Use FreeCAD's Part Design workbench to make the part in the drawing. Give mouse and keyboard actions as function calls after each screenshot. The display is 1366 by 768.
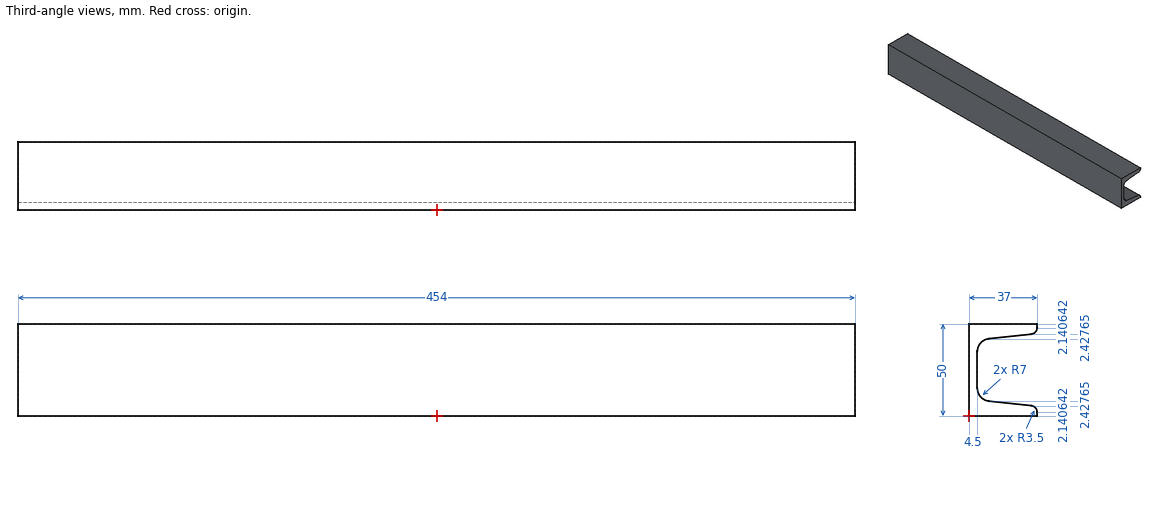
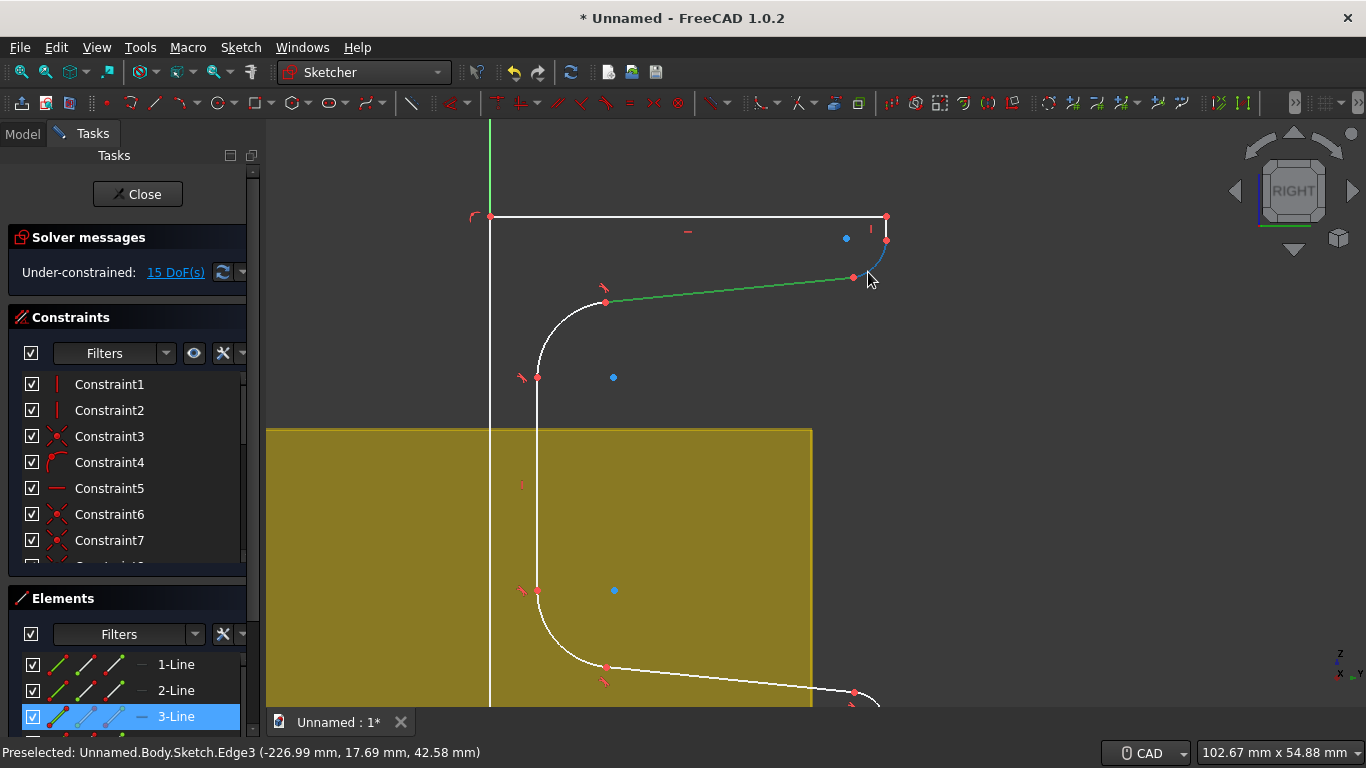
click(868, 272)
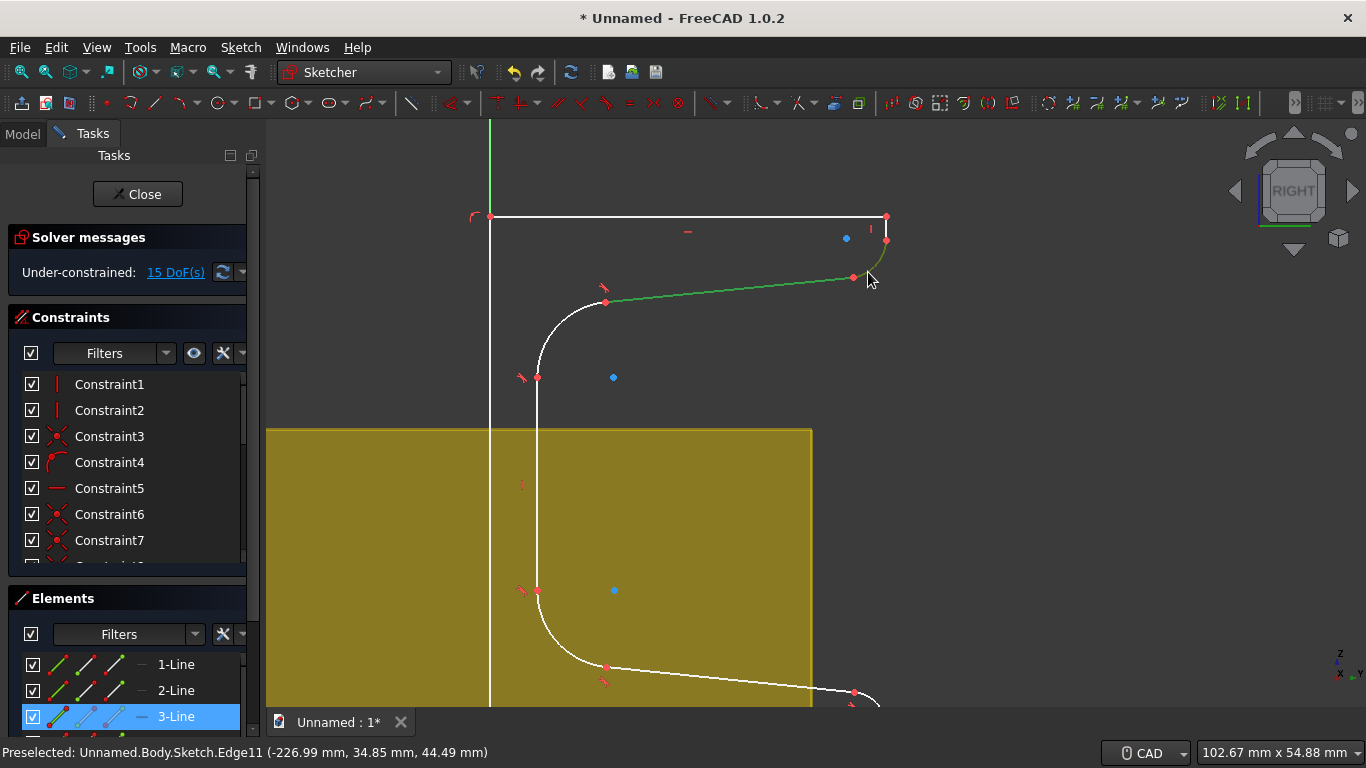
click(606, 104)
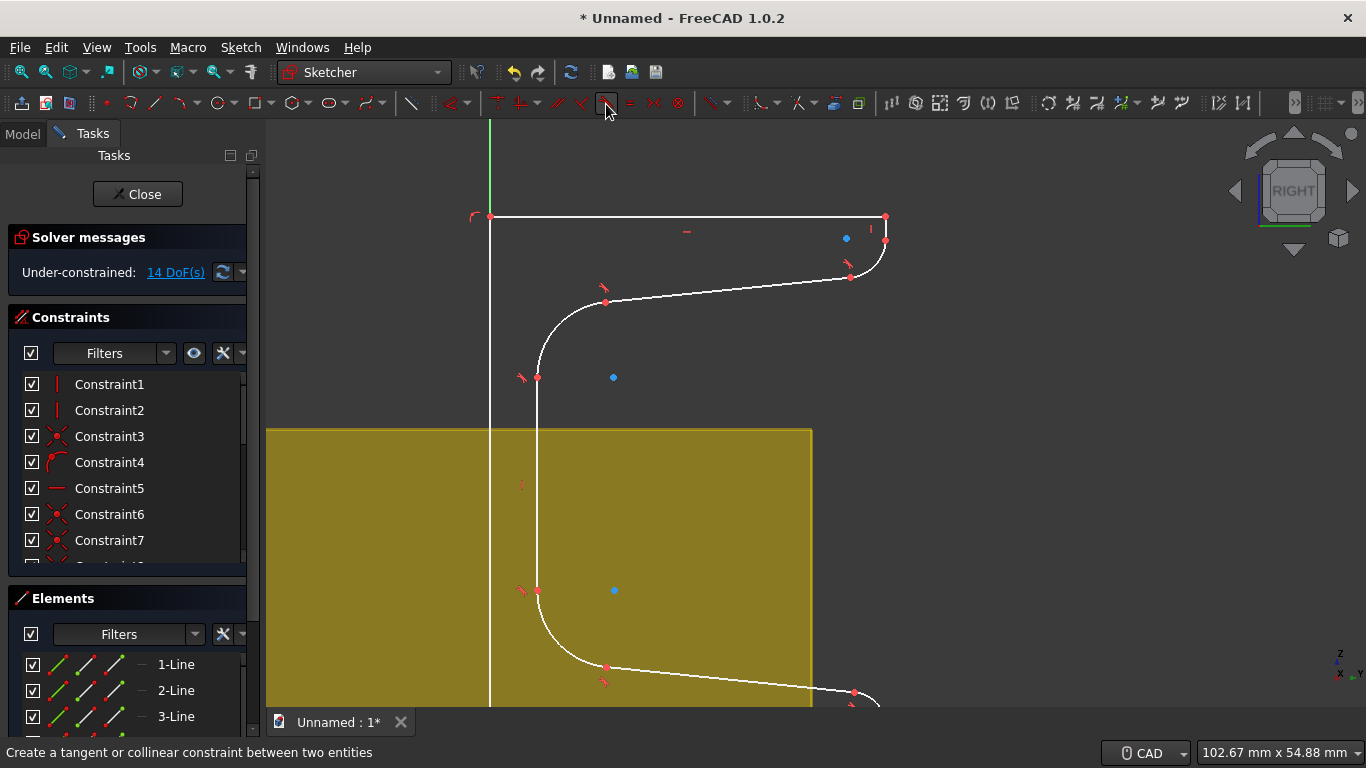
scroll(886, 231, up, 2)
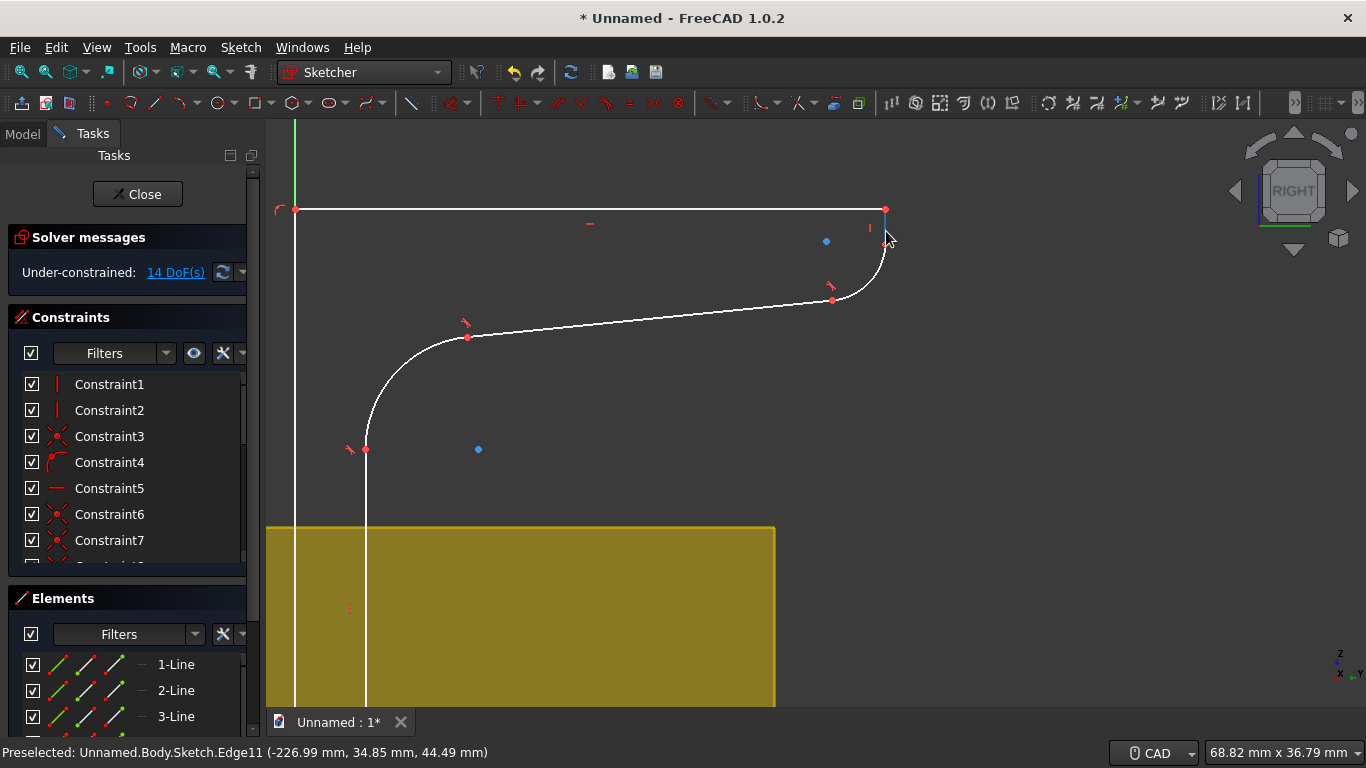
click(885, 231)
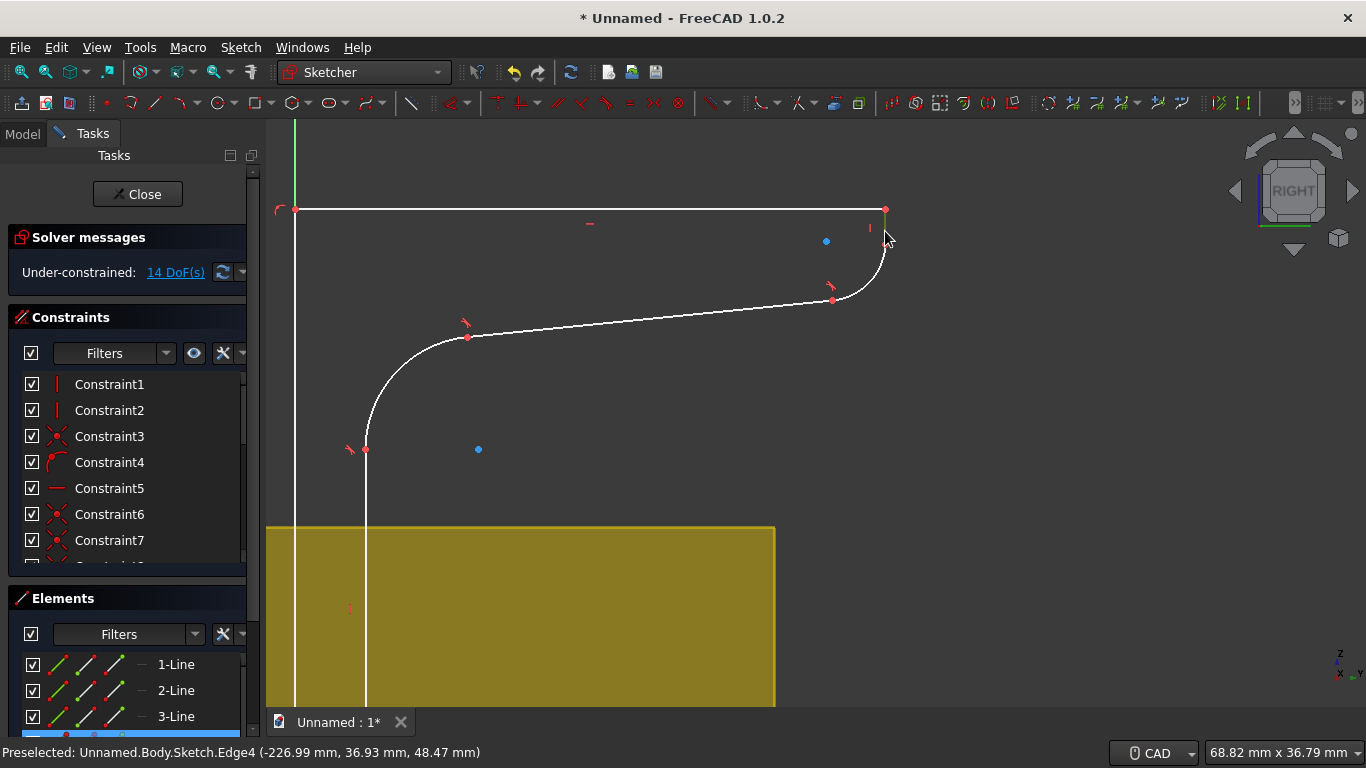
click(856, 293)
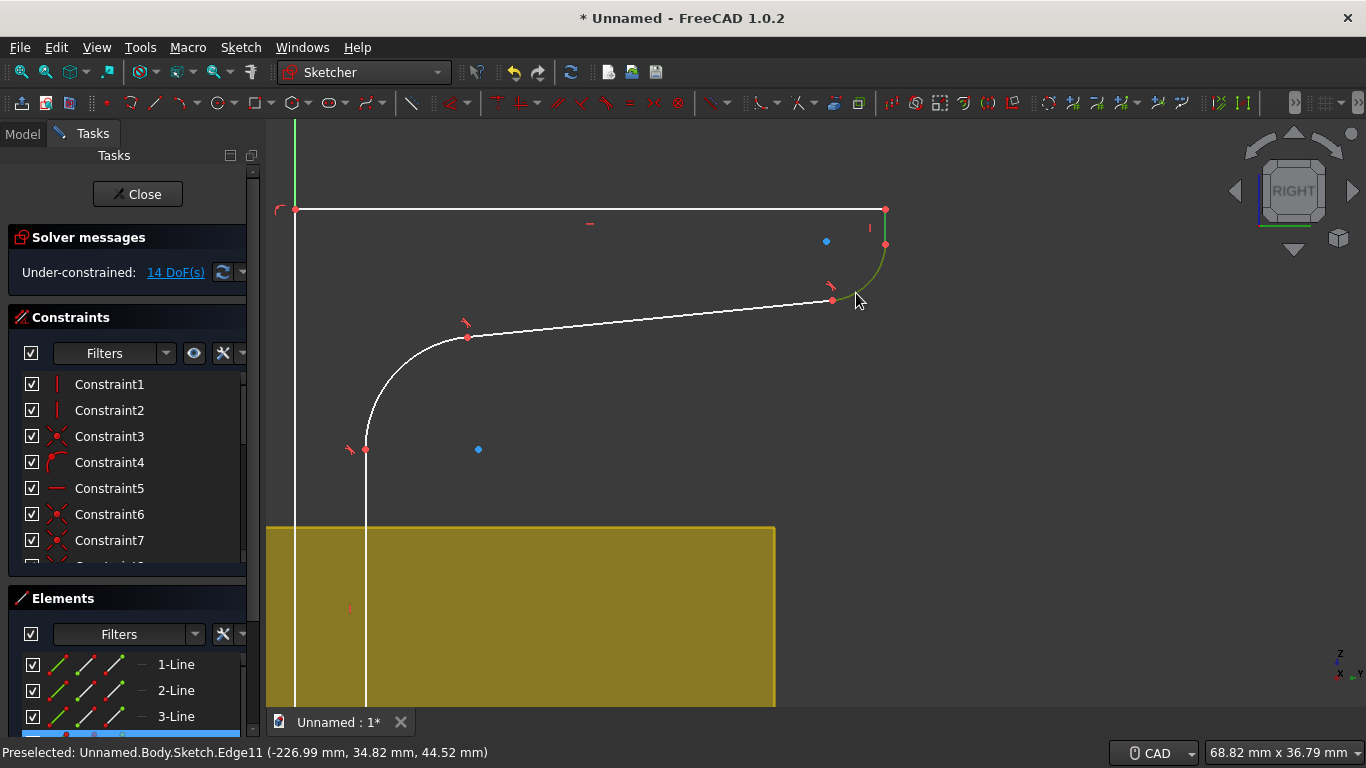
click(606, 104)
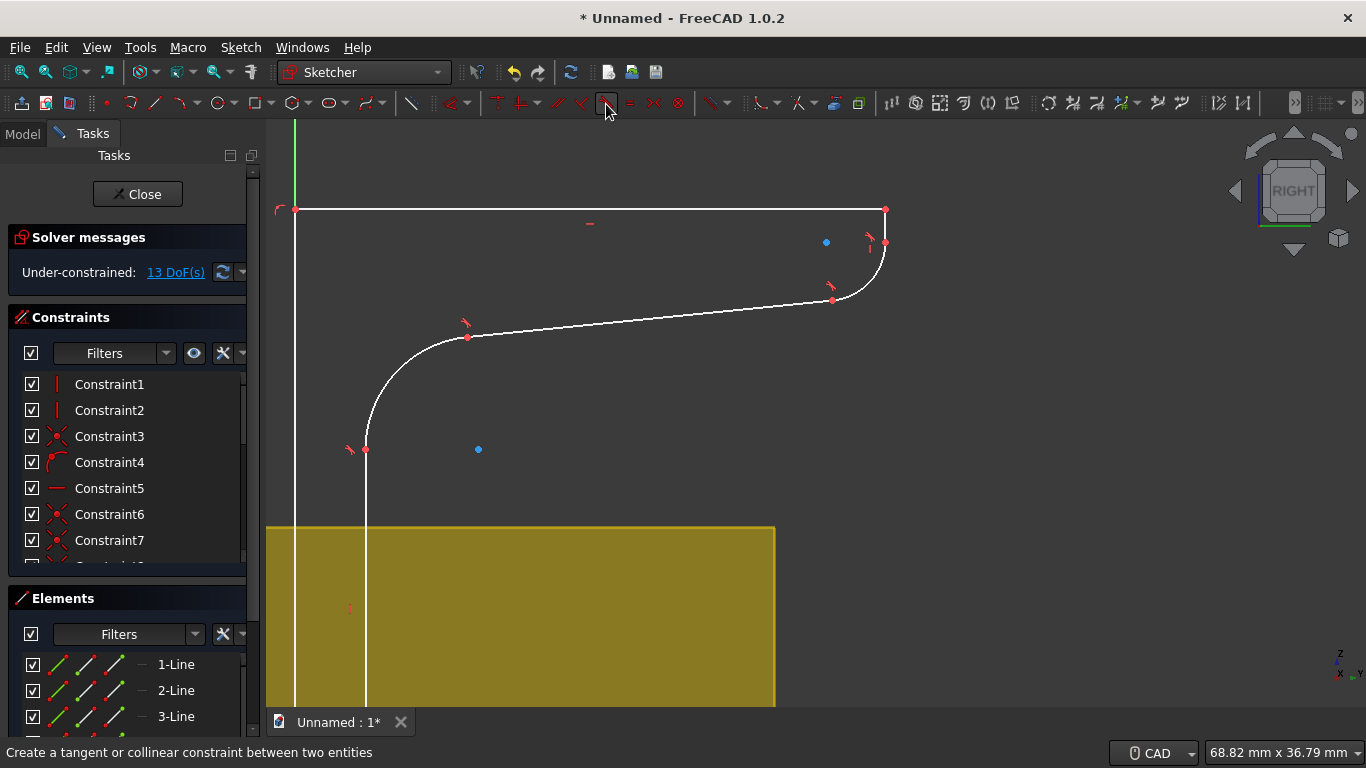
scroll(875, 255, down, 4)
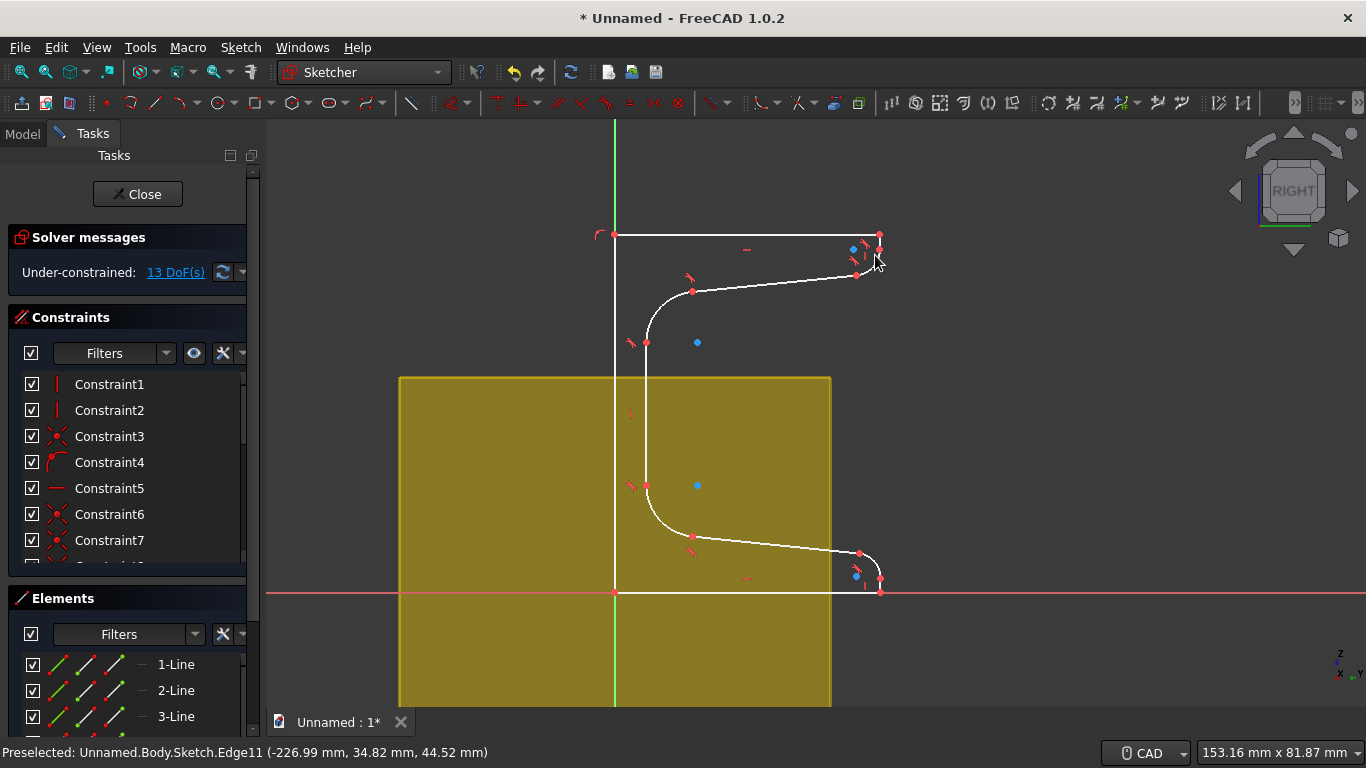
scroll(880, 589, up, 6)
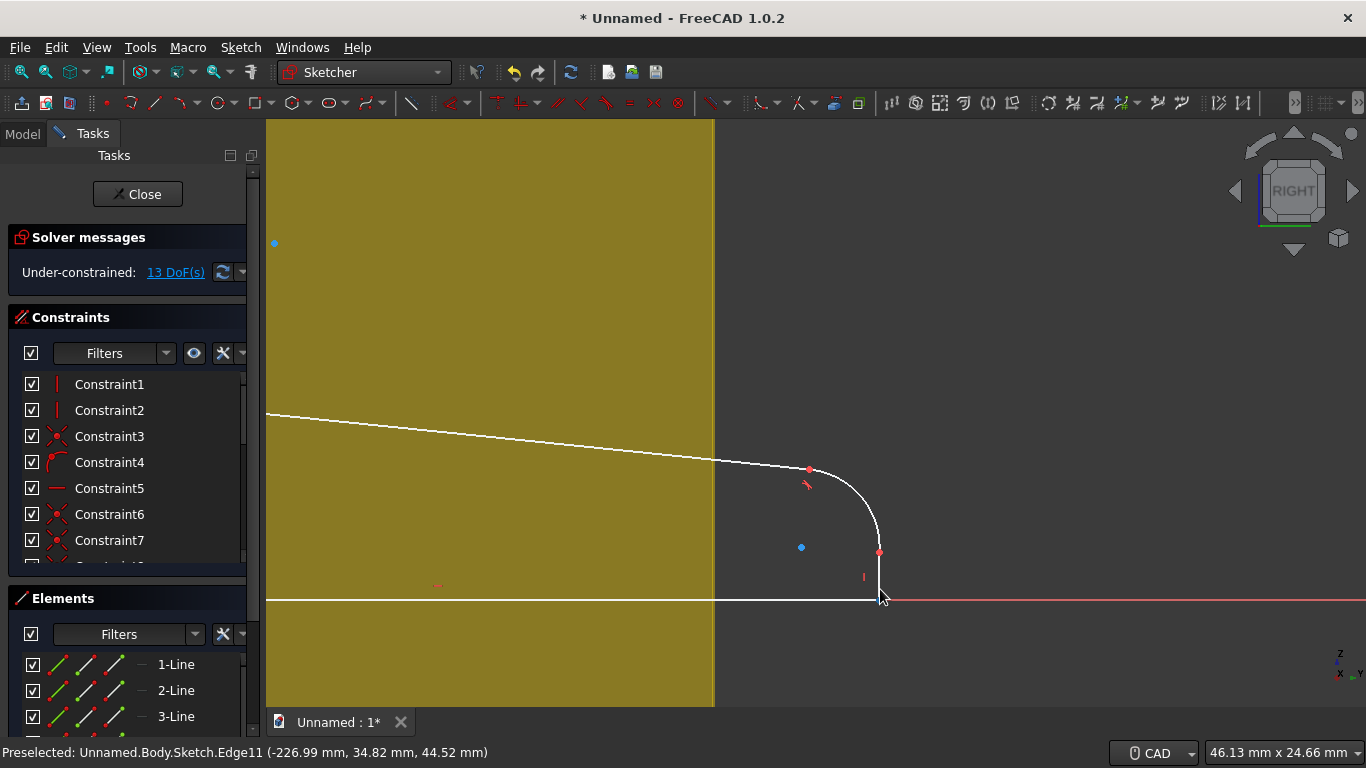
click(879, 586)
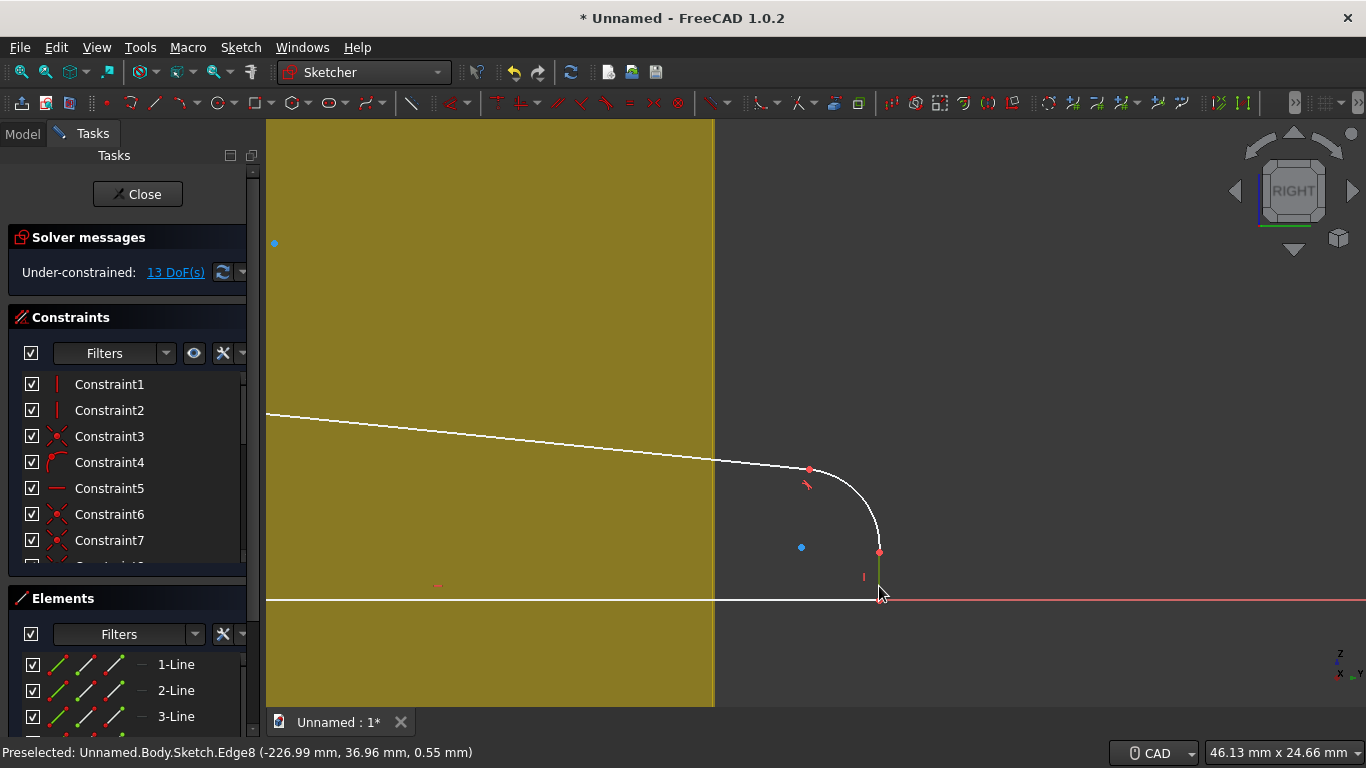
click(874, 517)